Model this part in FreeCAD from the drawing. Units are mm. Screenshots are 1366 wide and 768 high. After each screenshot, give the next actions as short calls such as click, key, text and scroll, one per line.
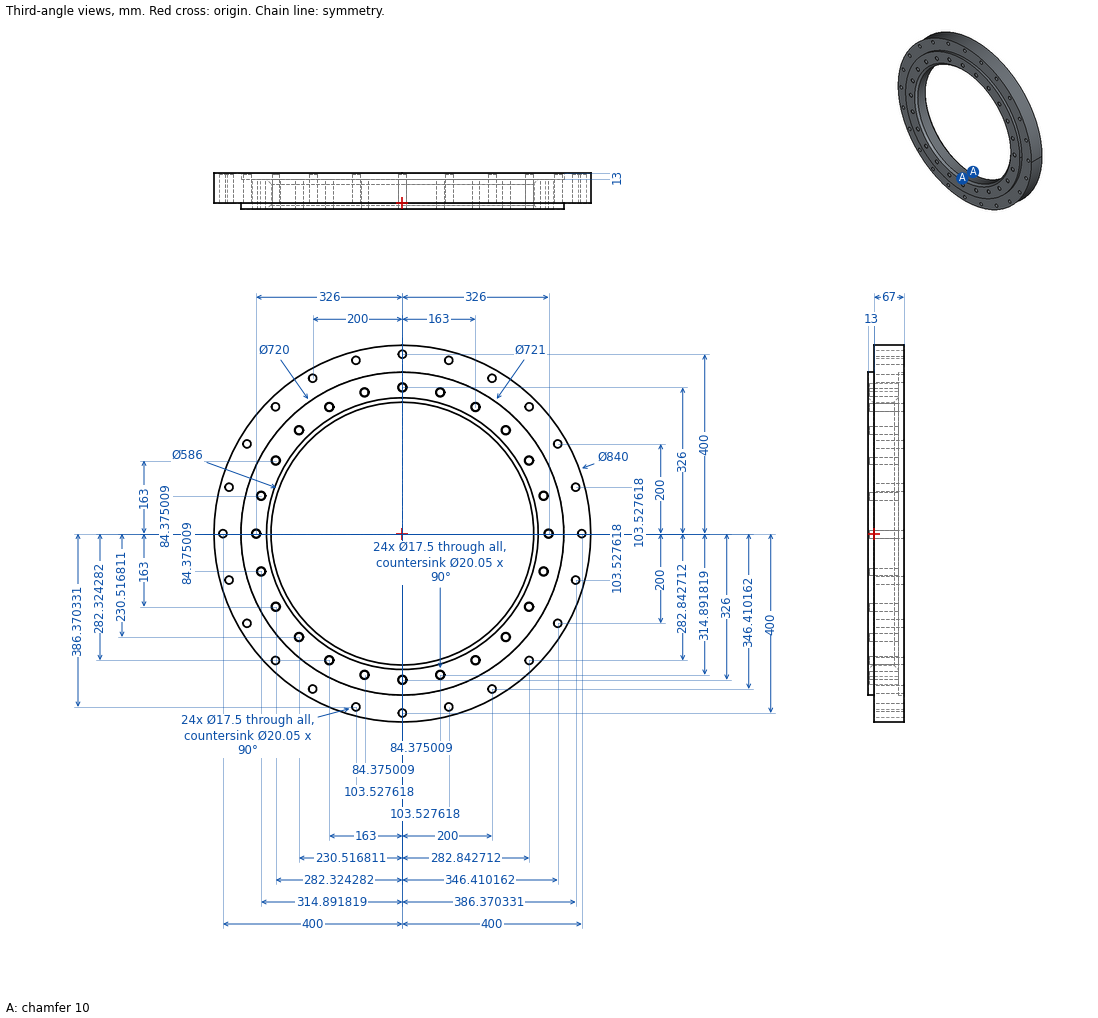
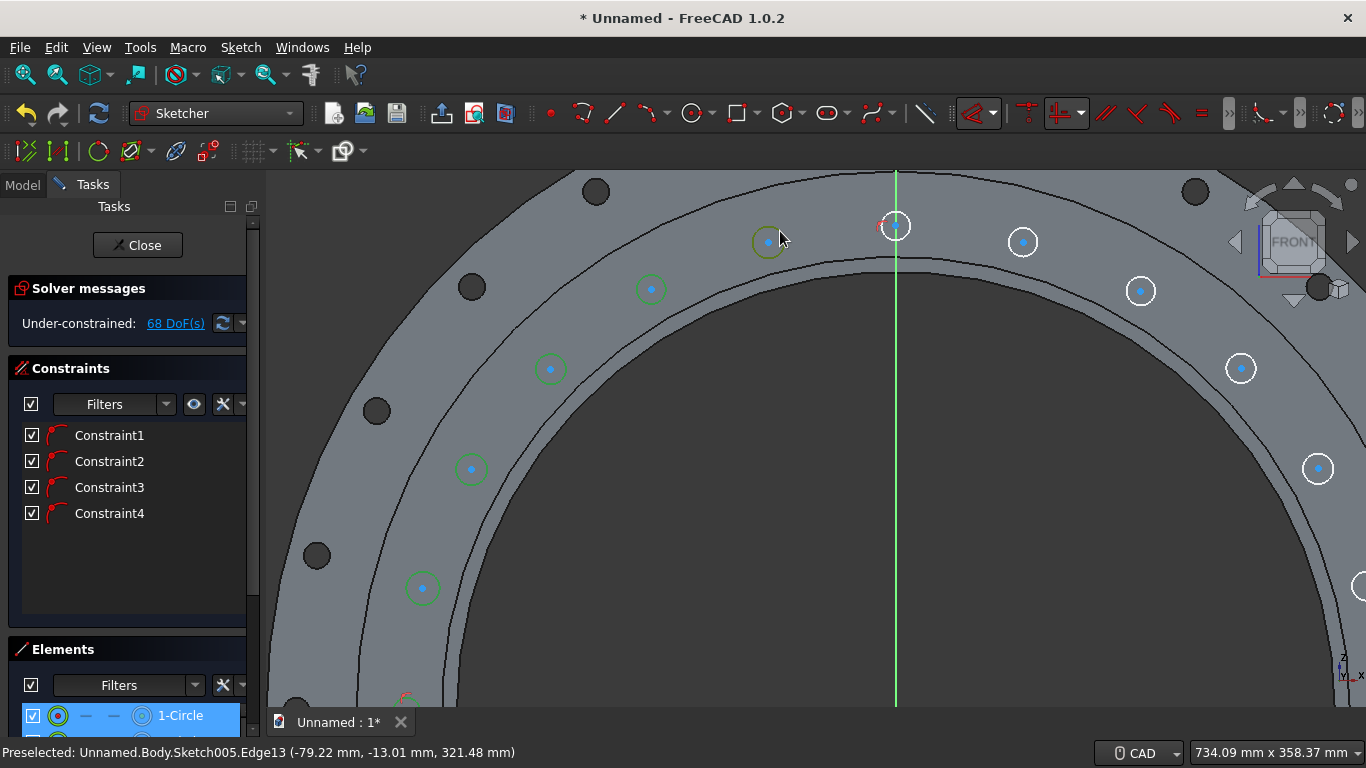
scroll(906, 216, up, 2)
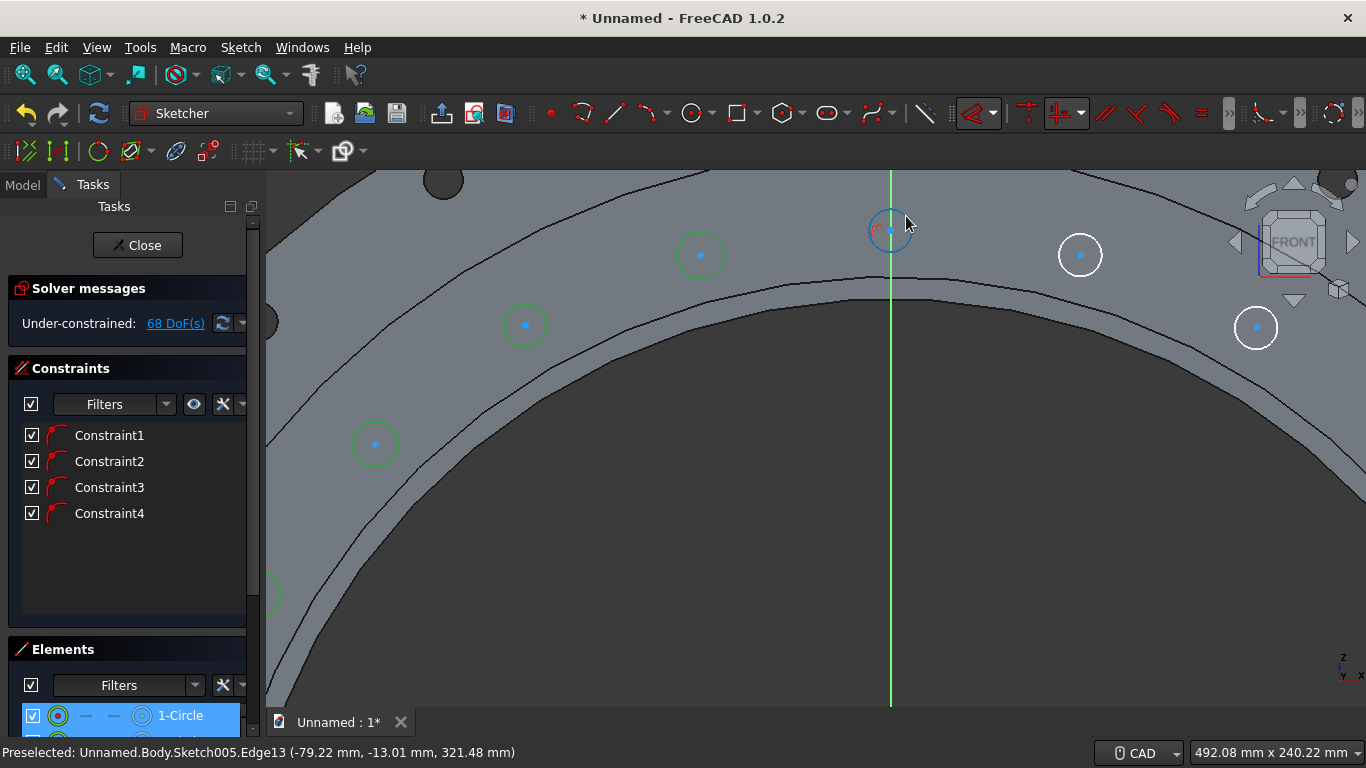
click(906, 216)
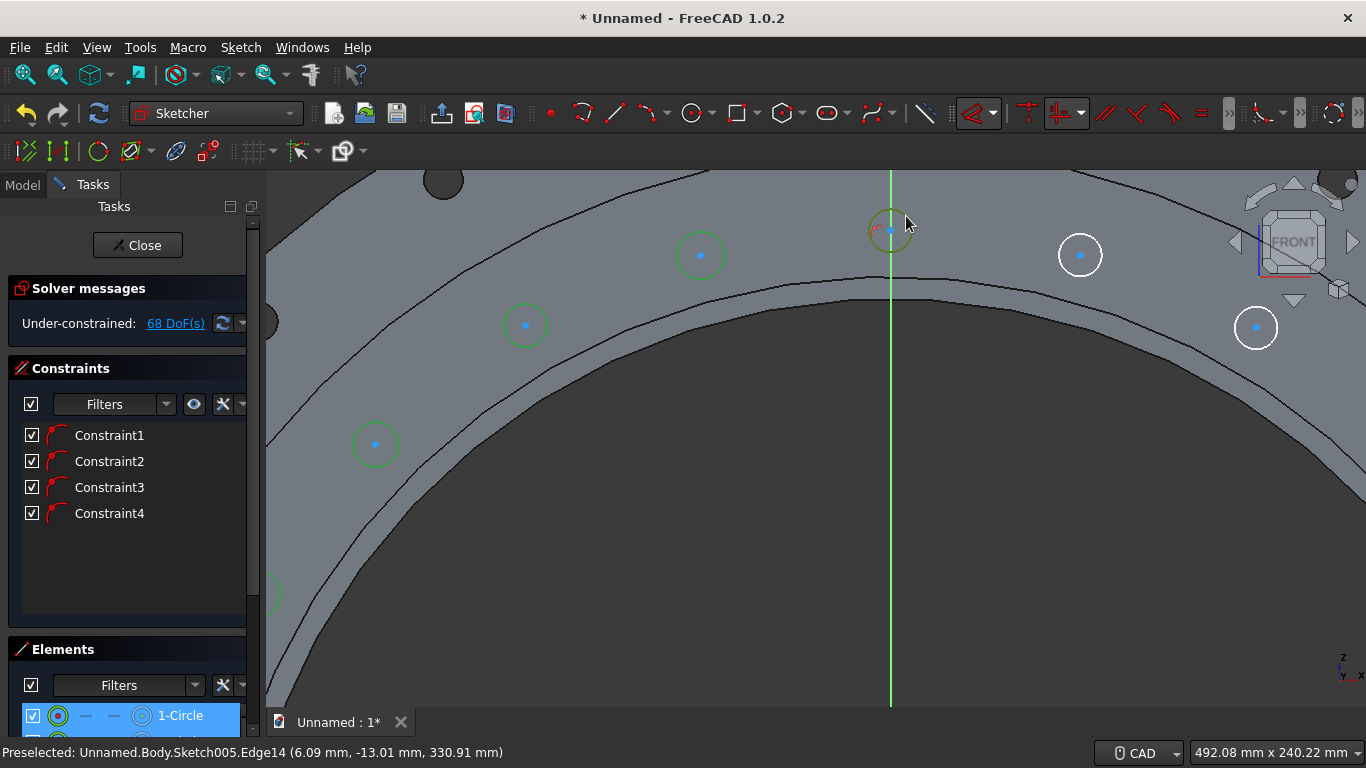
click(1095, 240)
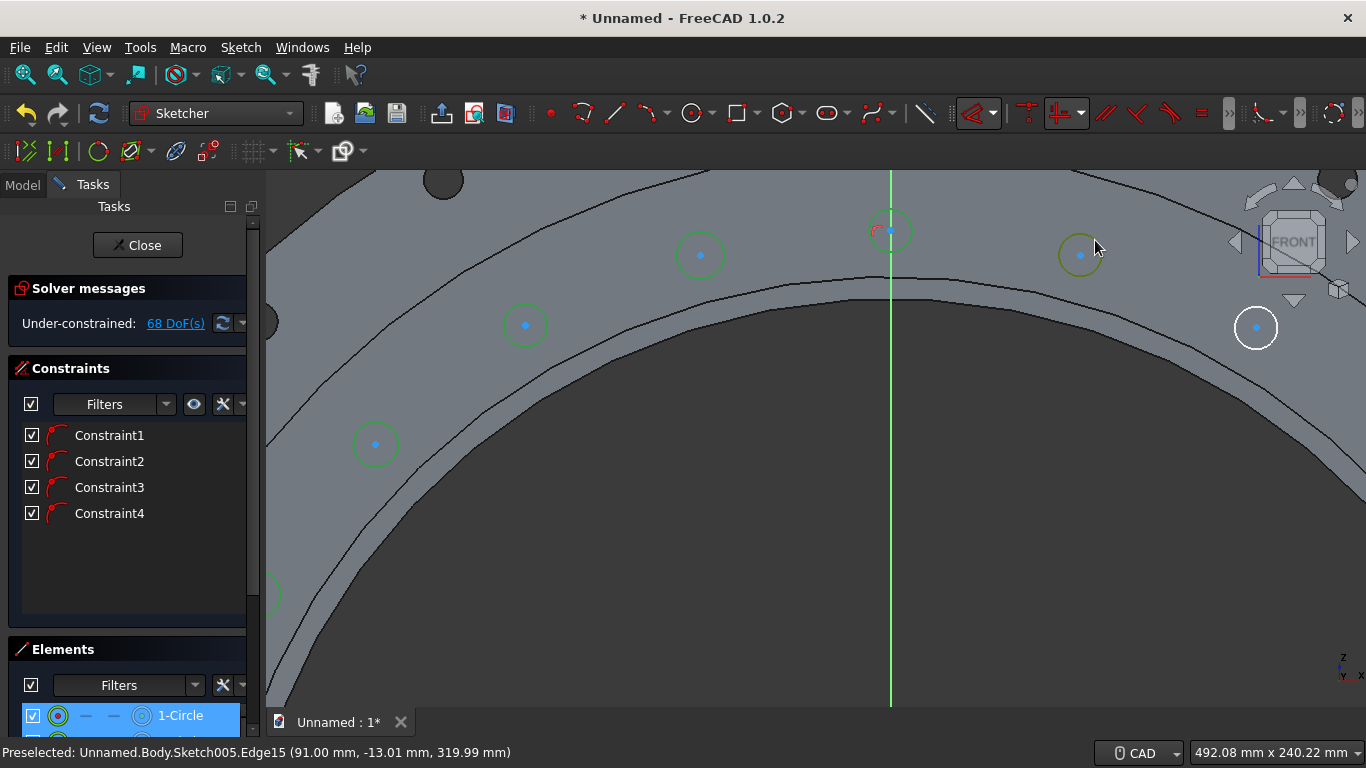
scroll(701, 270, down, 7)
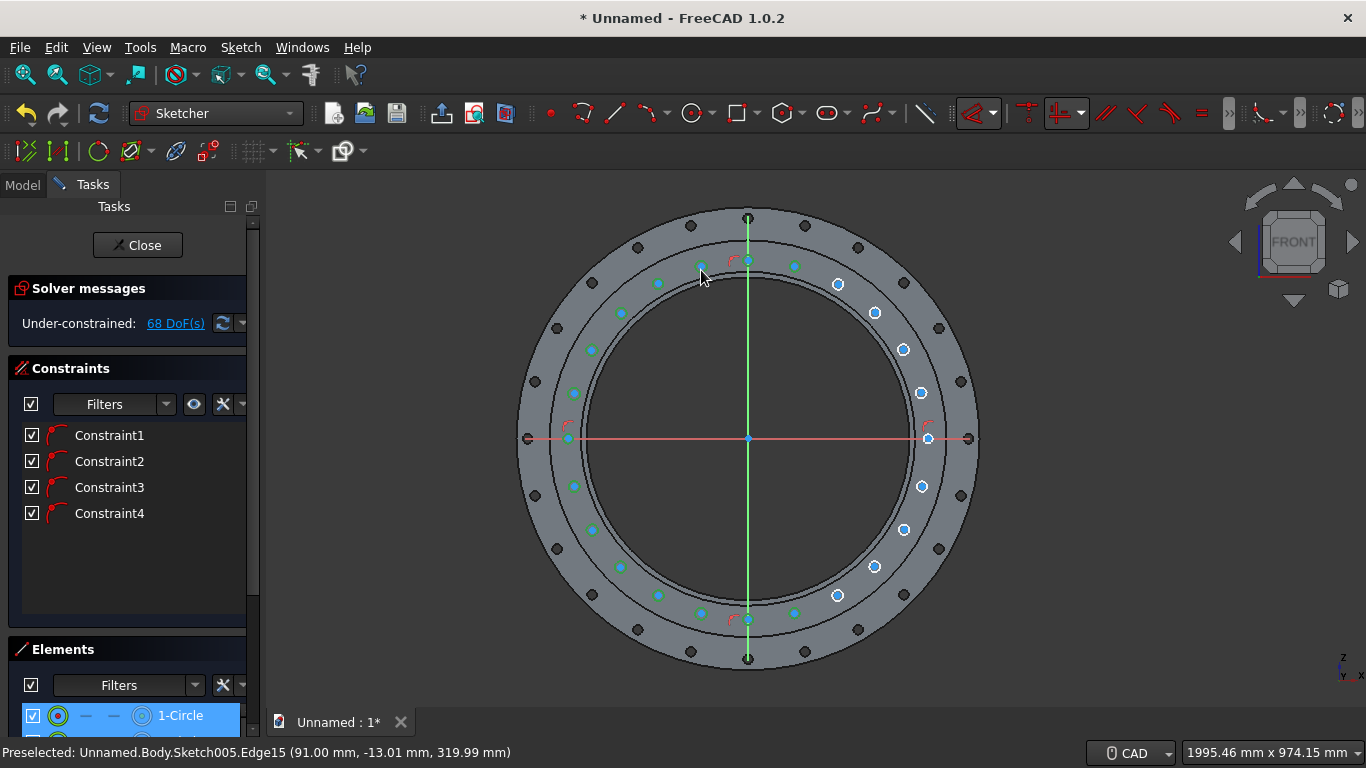
scroll(842, 281, up, 5)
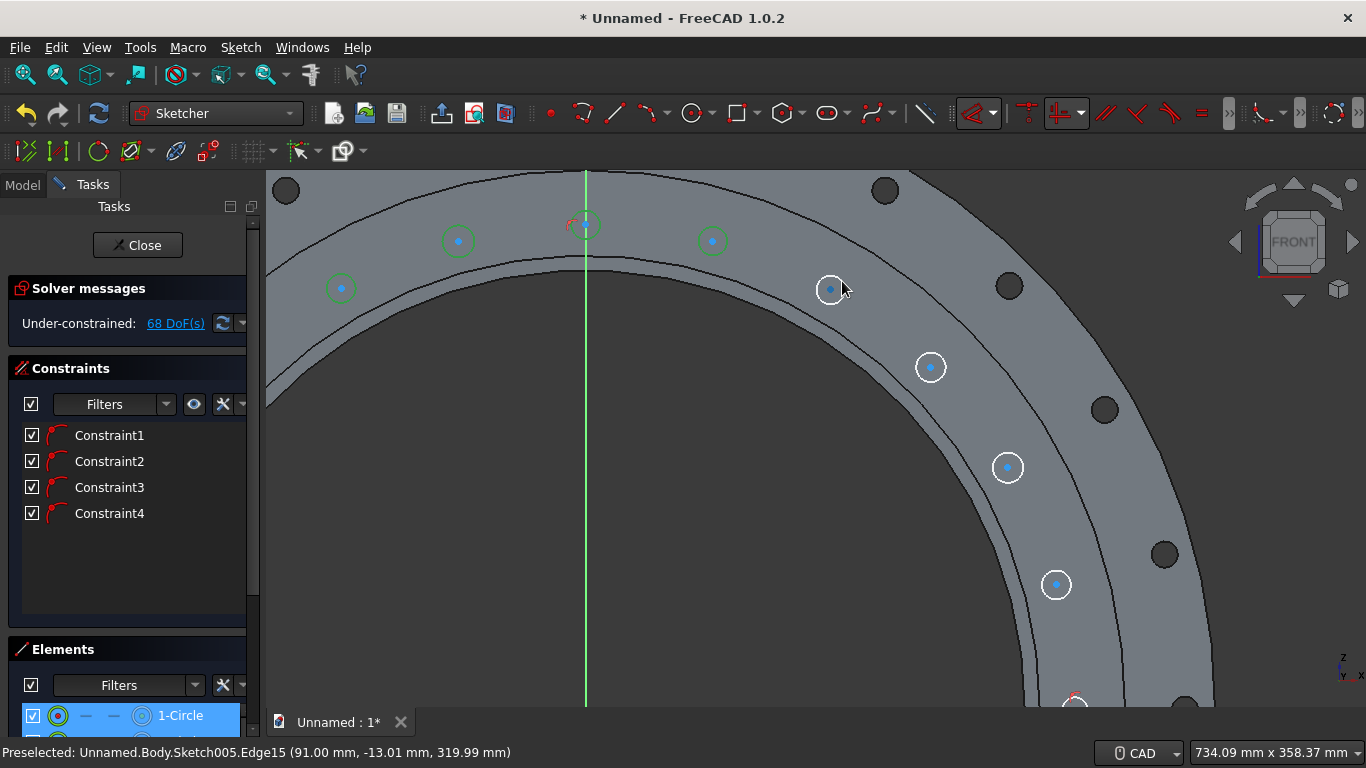
click(841, 280)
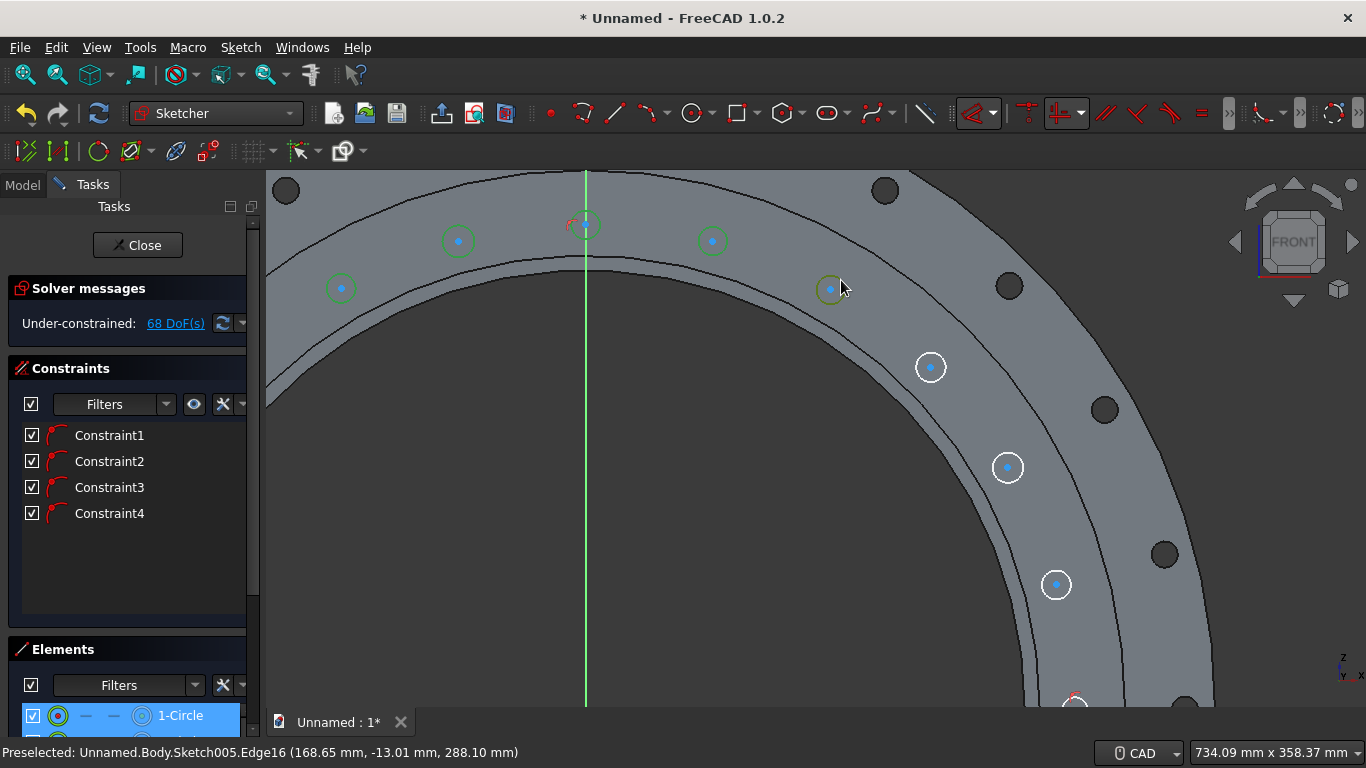
click(941, 357)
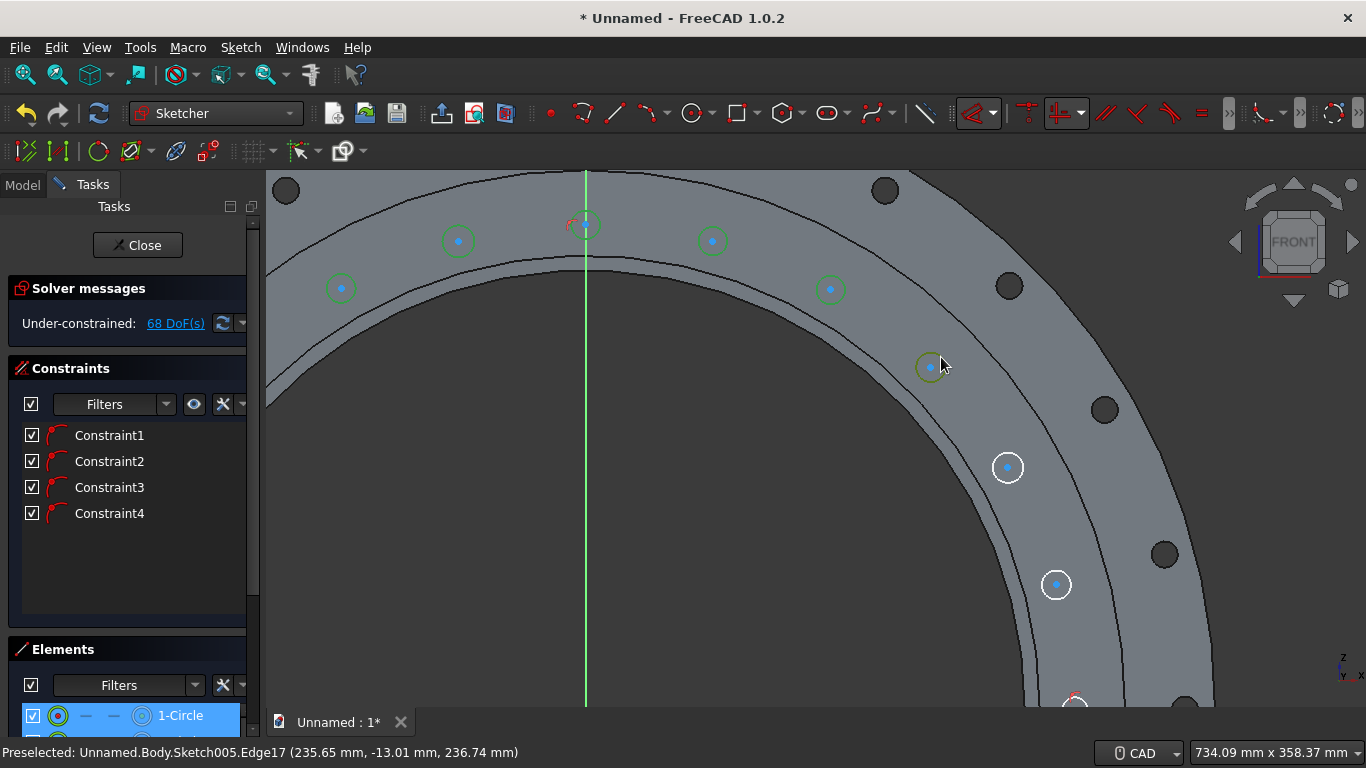
click(1019, 457)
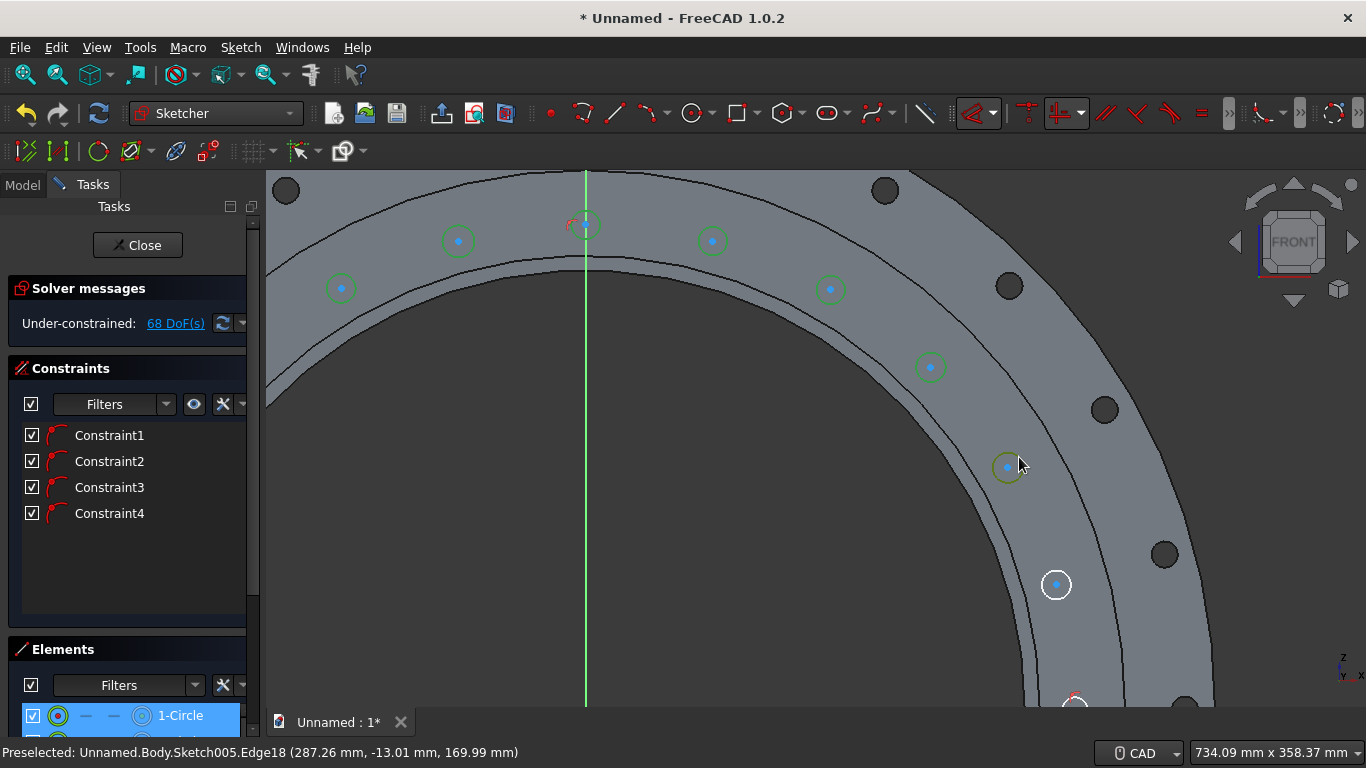
click(1067, 575)